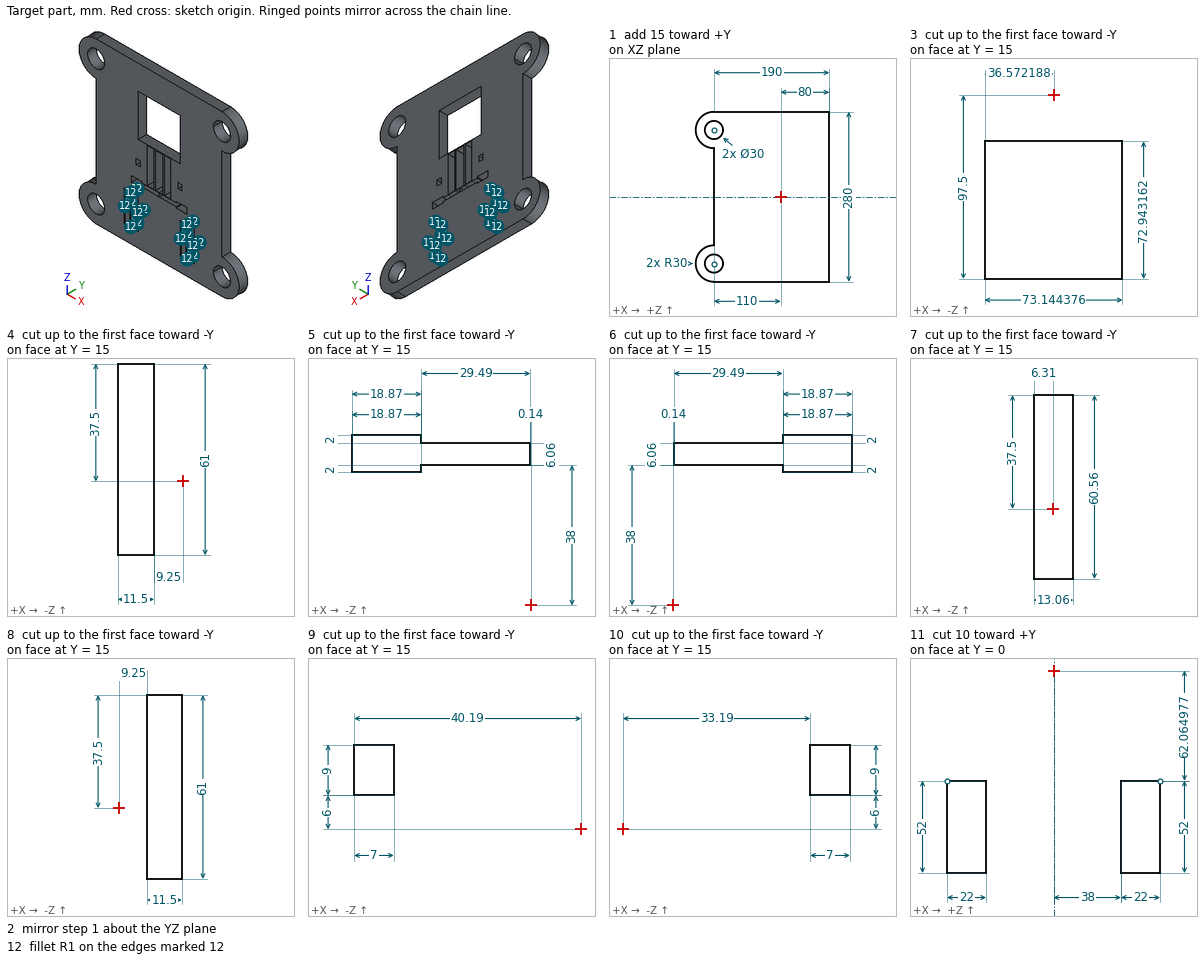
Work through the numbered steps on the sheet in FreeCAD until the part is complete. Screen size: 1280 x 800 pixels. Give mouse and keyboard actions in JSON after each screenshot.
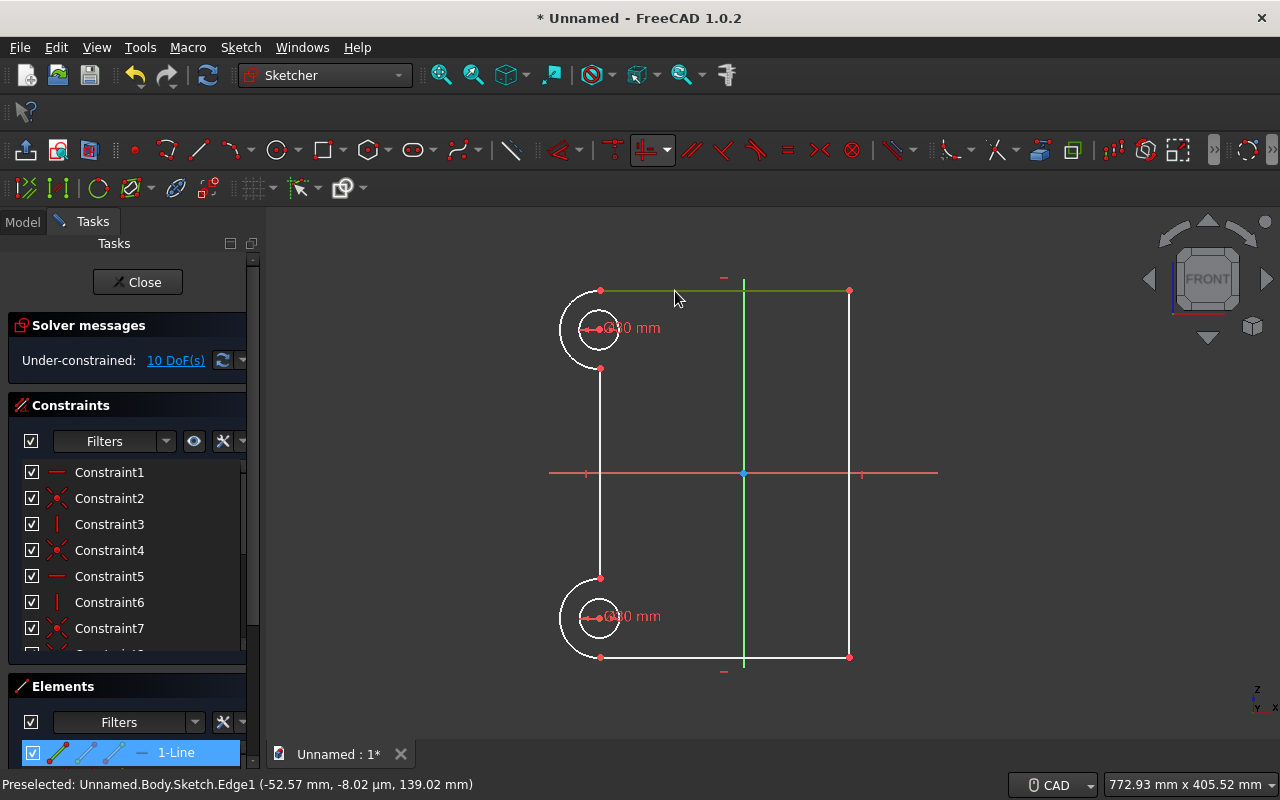
{"action": "left_click", "coordinate": [568, 307]}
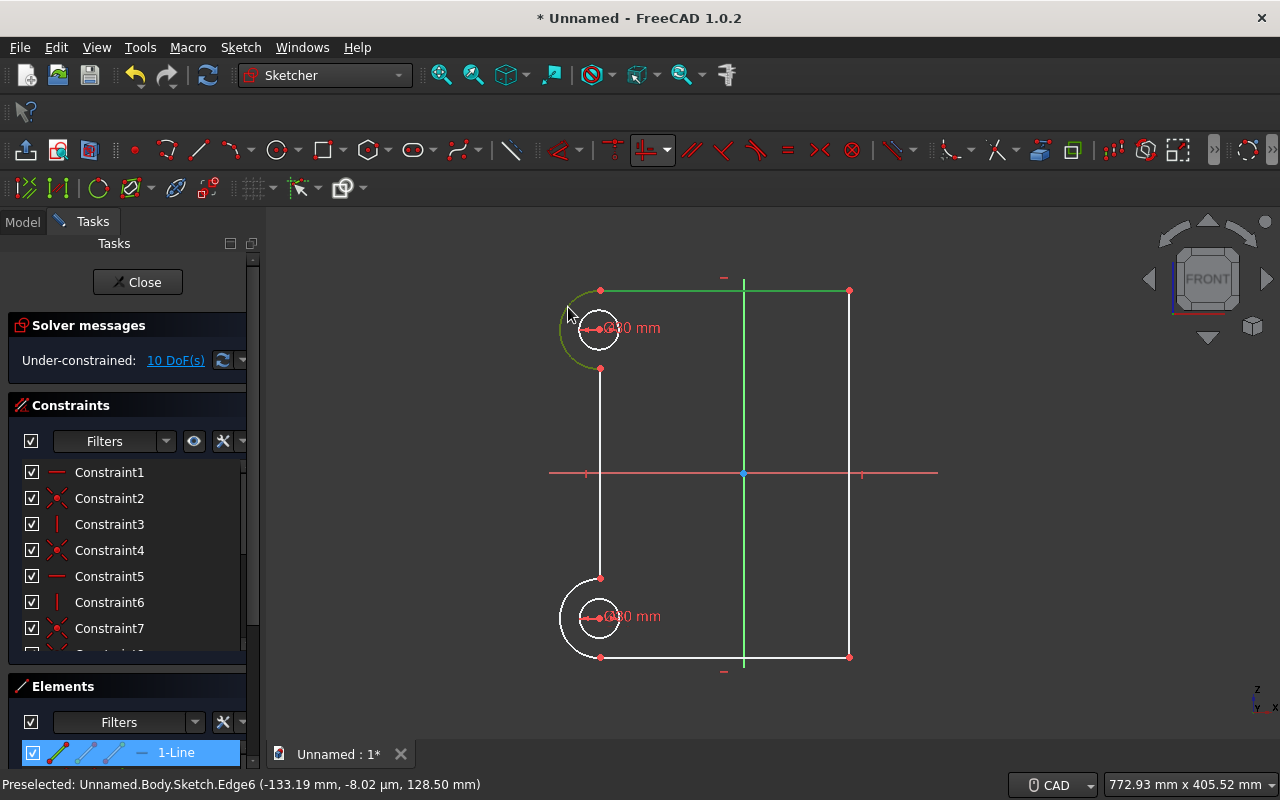
{"action": "left_click", "coordinate": [756, 150]}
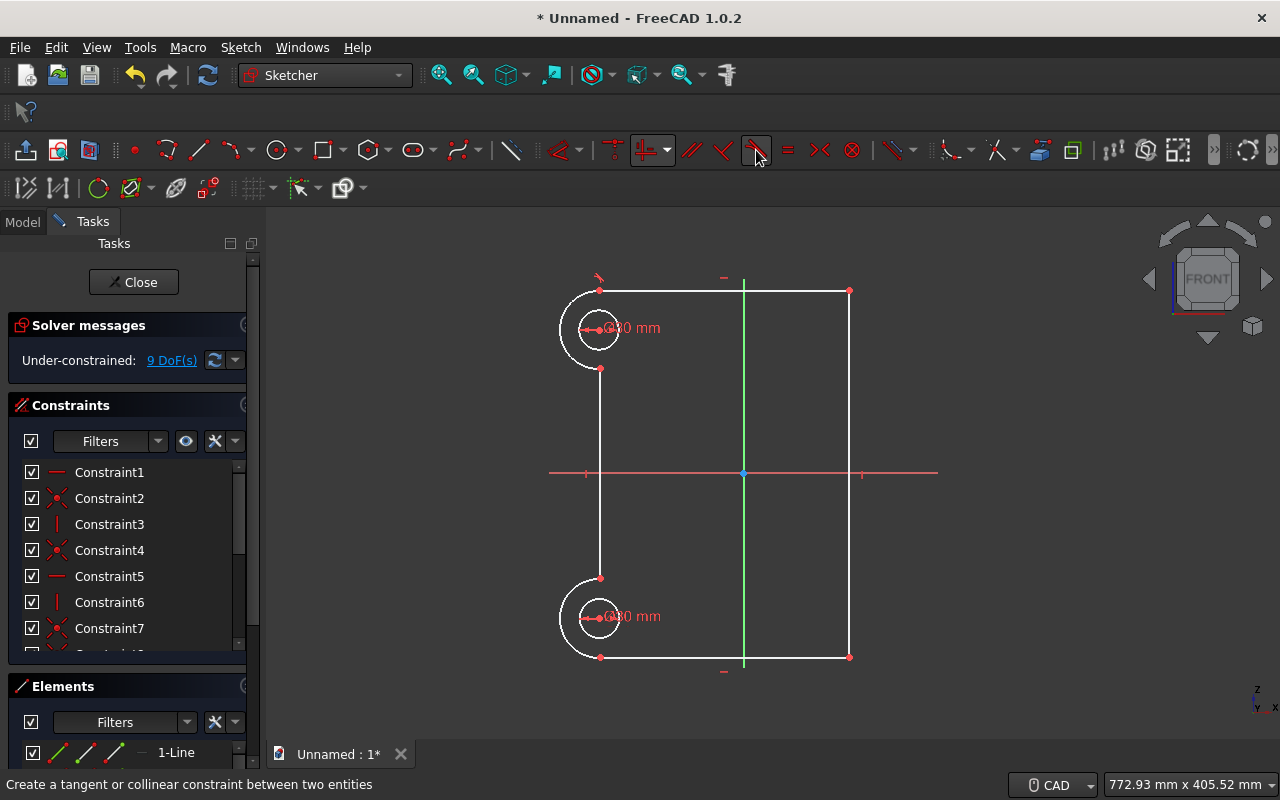
{"action": "left_click", "coordinate": [774, 658]}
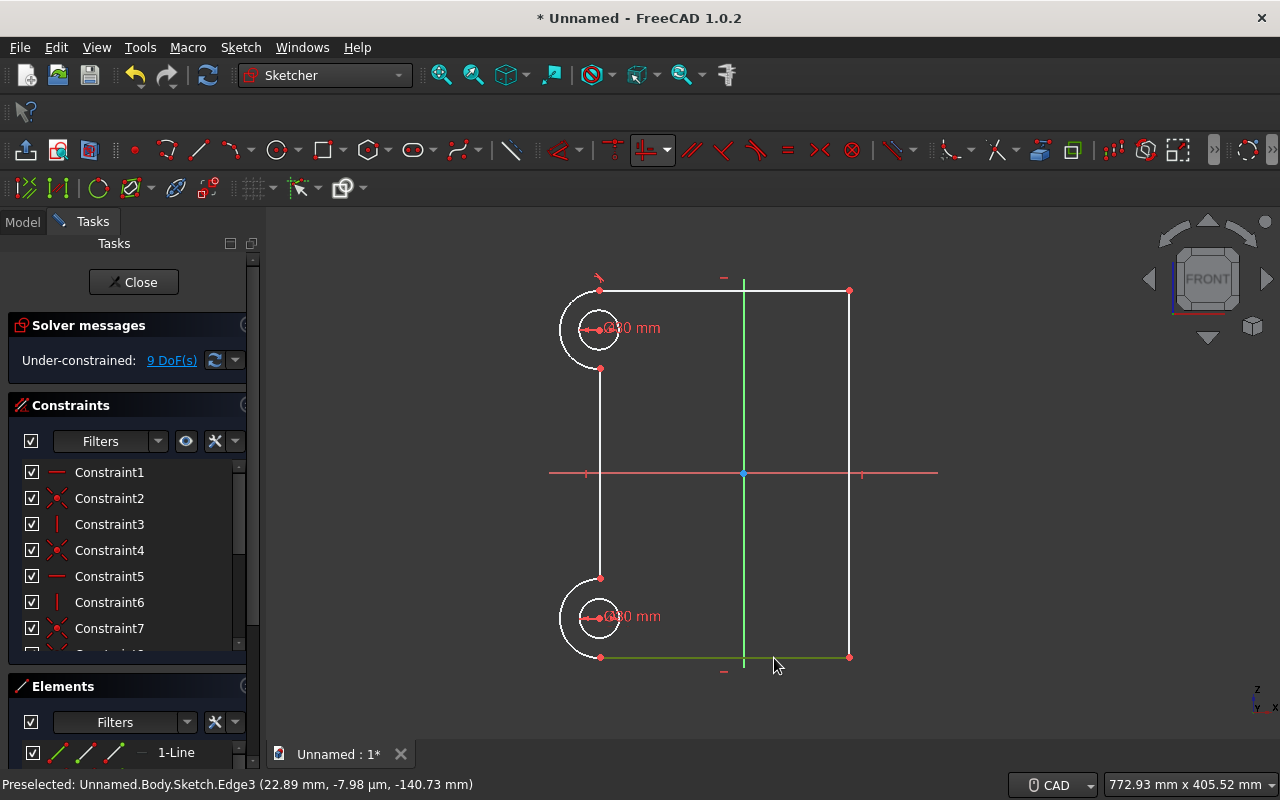
{"action": "left_click", "coordinate": [568, 595]}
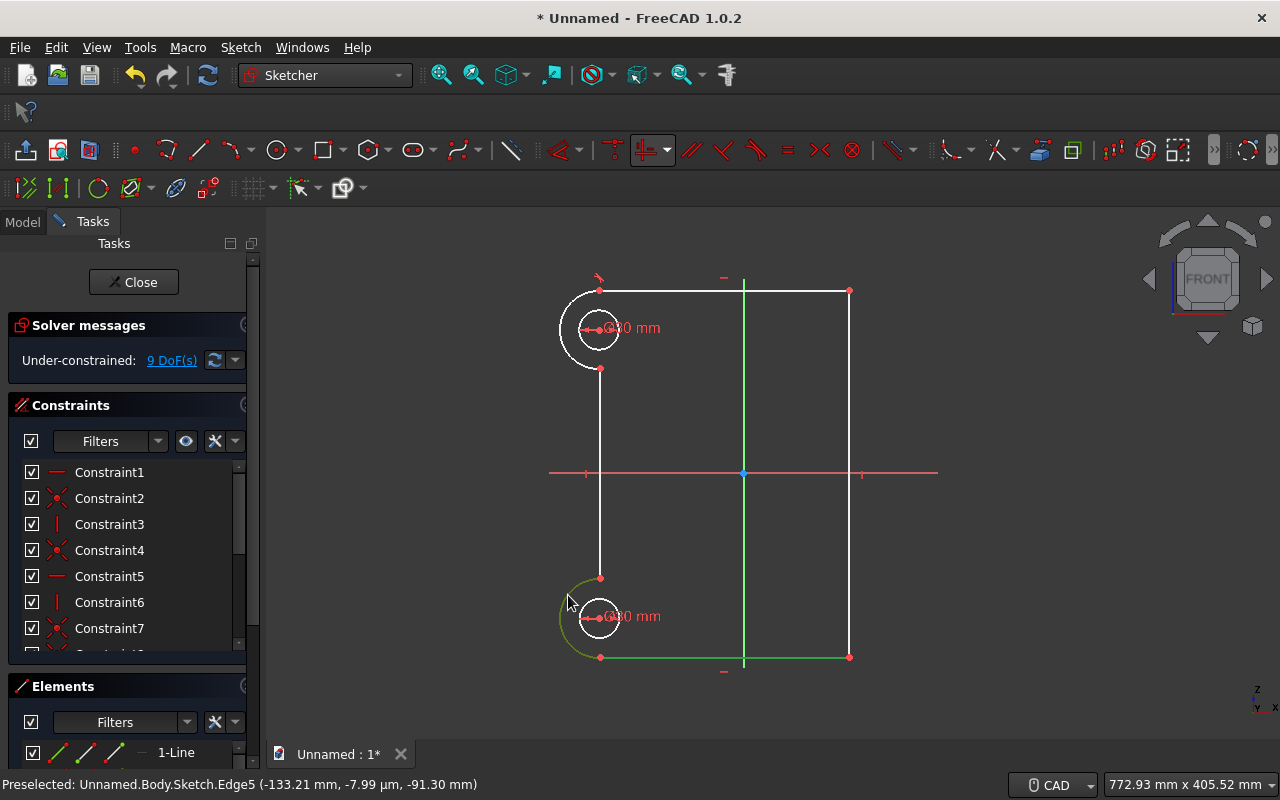
{"action": "left_click", "coordinate": [756, 150]}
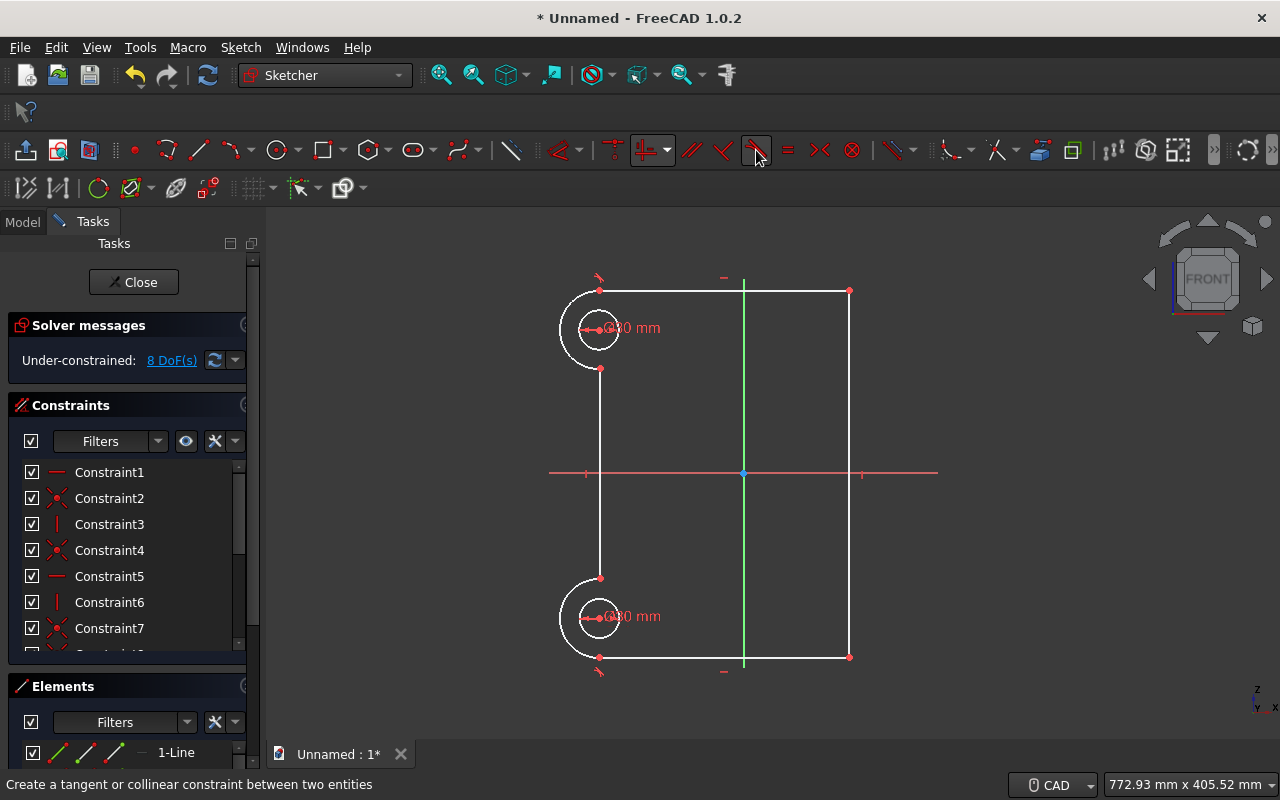
{"action": "left_click", "coordinate": [568, 595]}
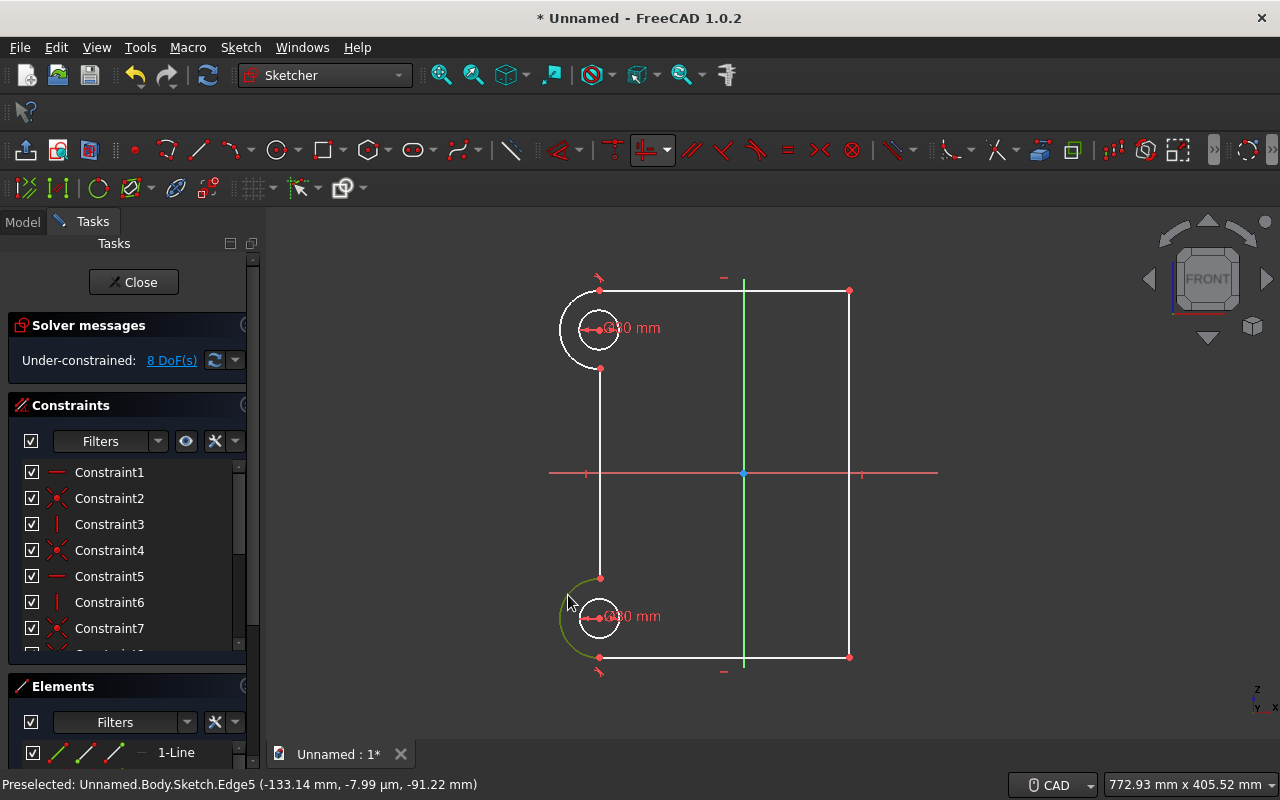
{"action": "left_click", "coordinate": [567, 307]}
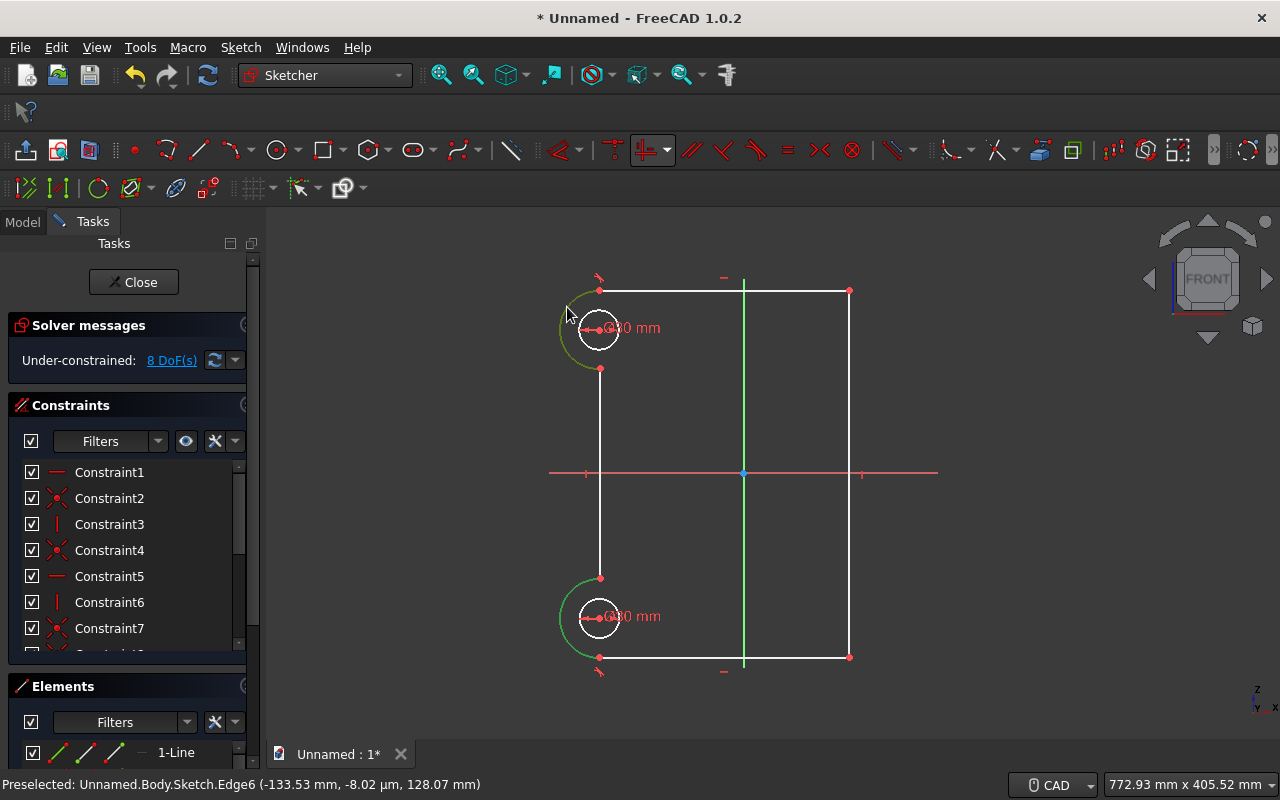
{"action": "left_click", "coordinate": [788, 150]}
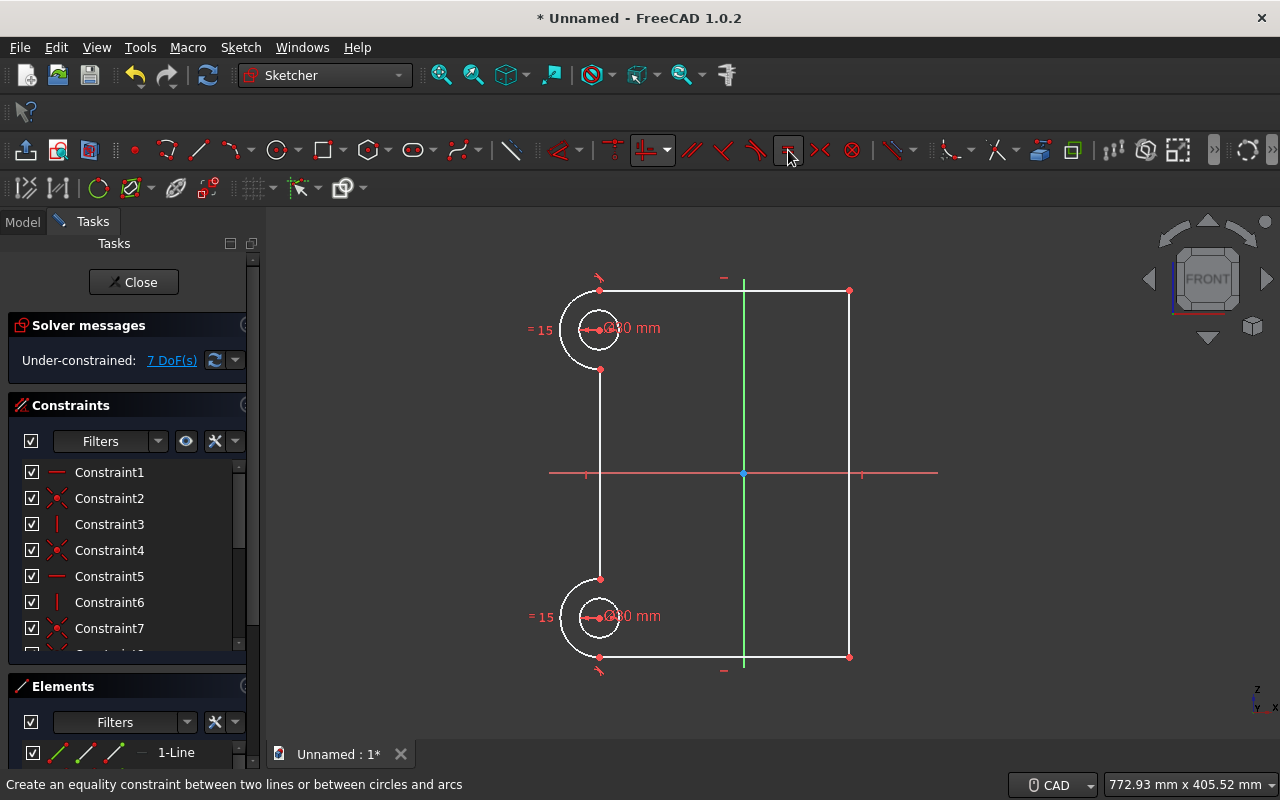
{"action": "left_click", "coordinate": [600, 618]}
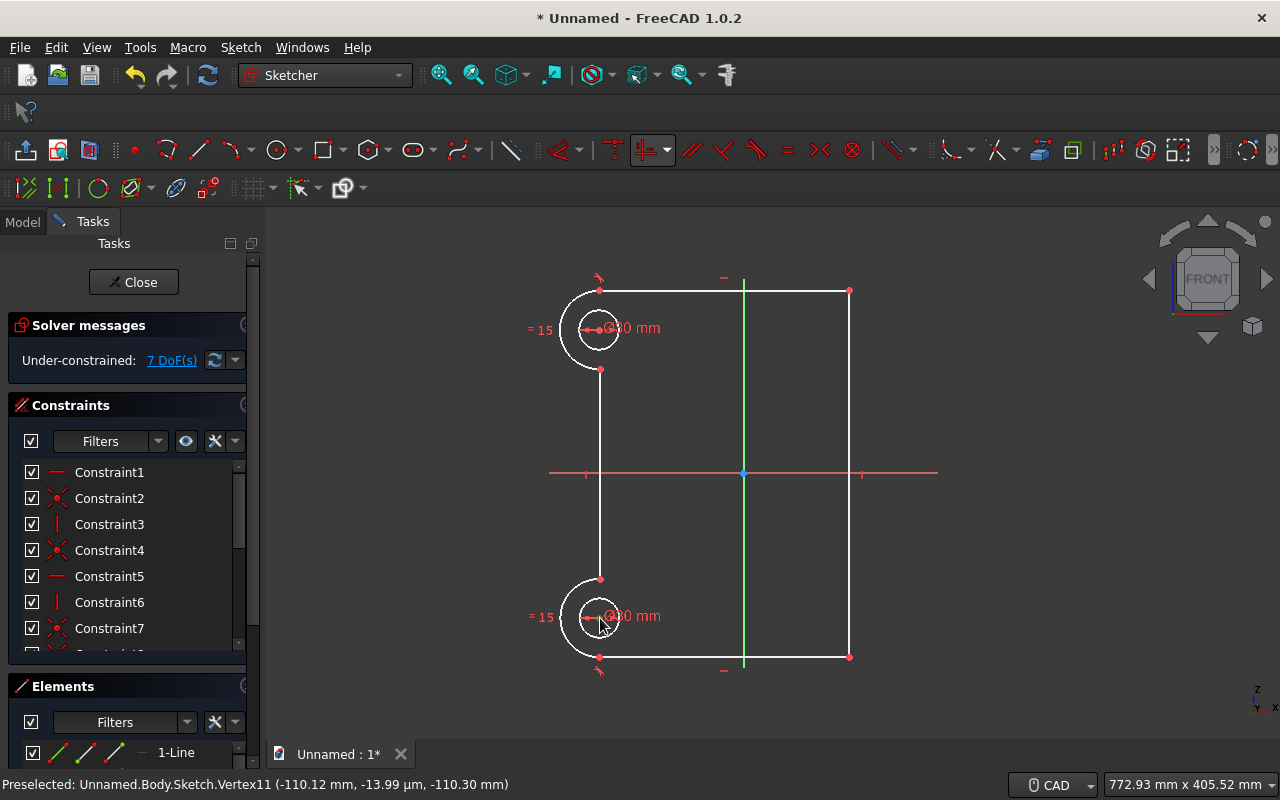
{"action": "left_click", "coordinate": [599, 330]}